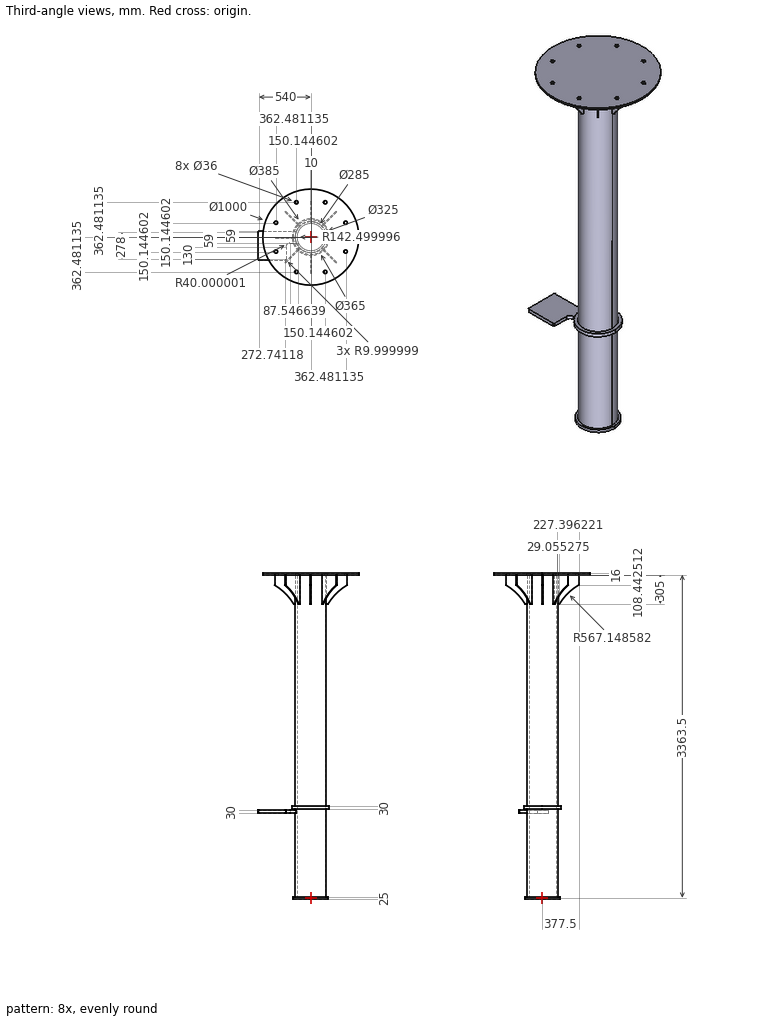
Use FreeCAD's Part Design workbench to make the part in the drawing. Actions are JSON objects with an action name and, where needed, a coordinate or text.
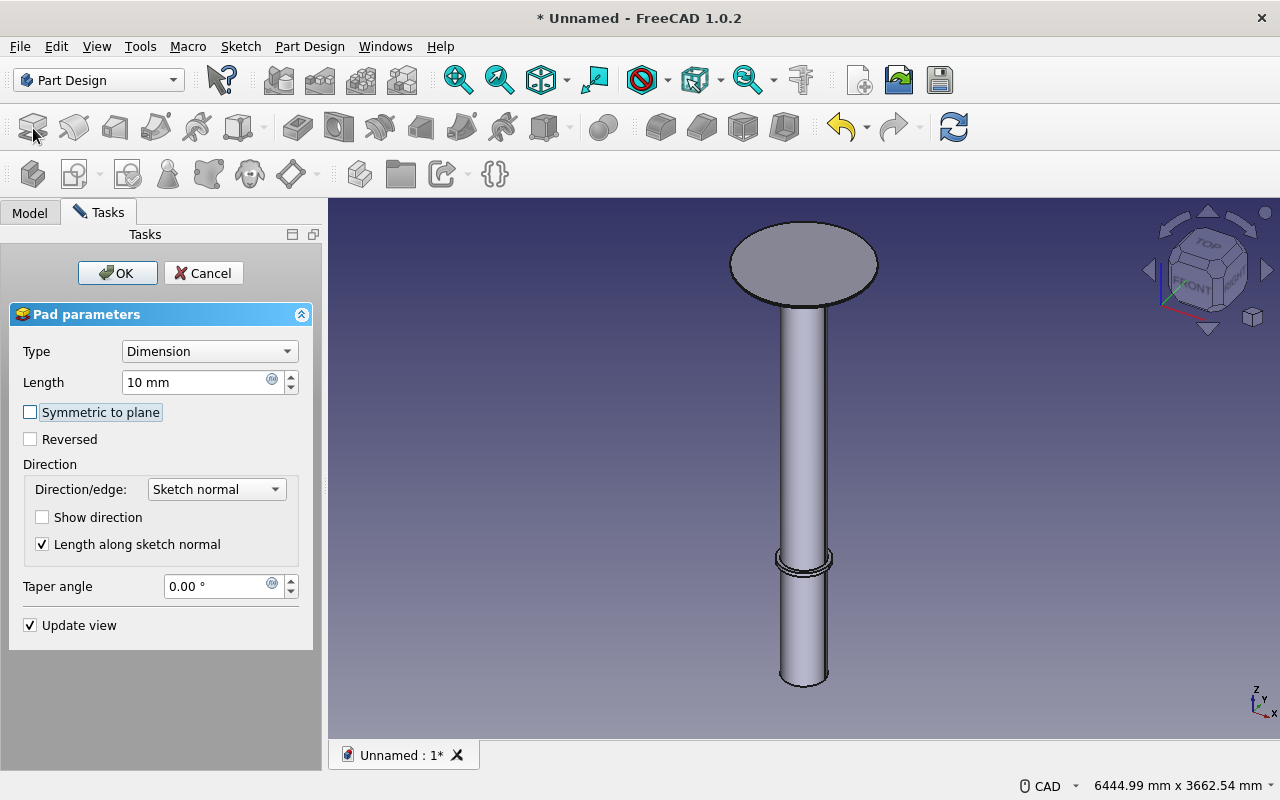
{"action": "left_click", "coordinate": [31, 412]}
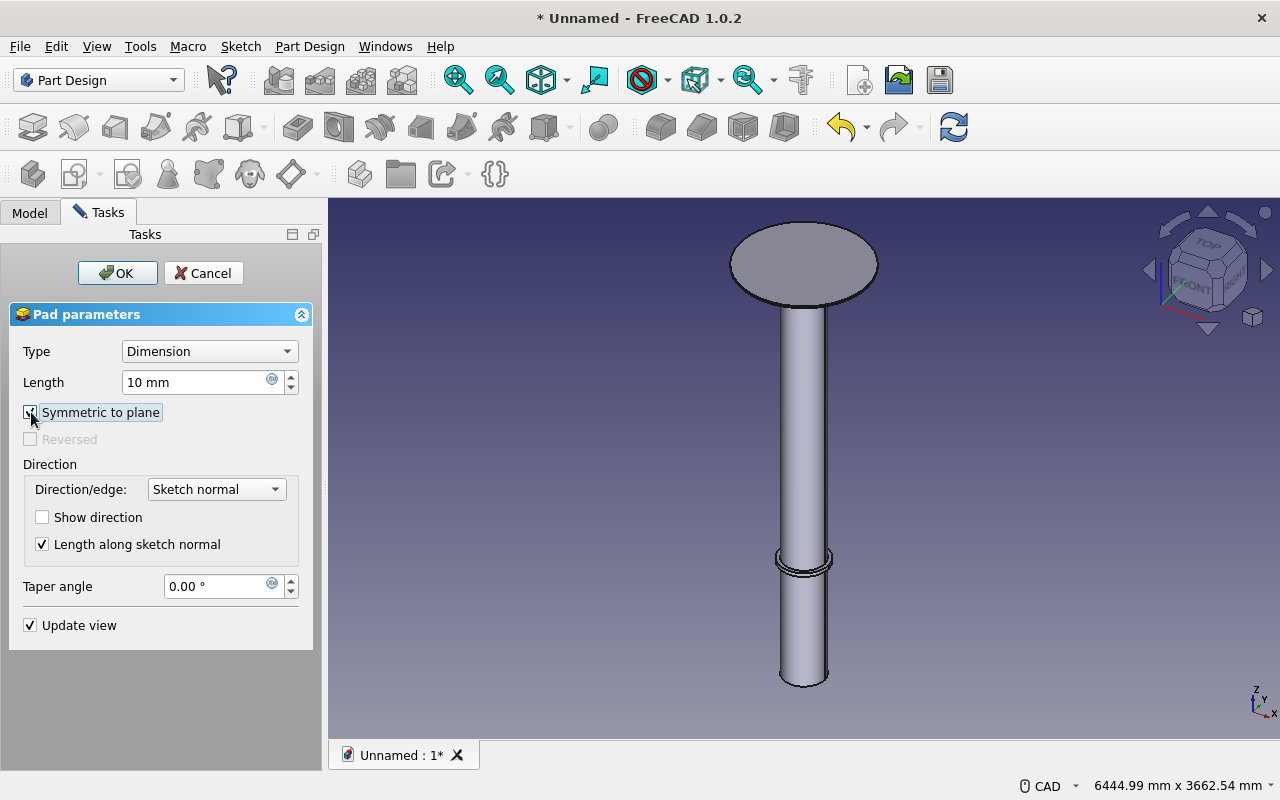
{"action": "left_click", "coordinate": [118, 273]}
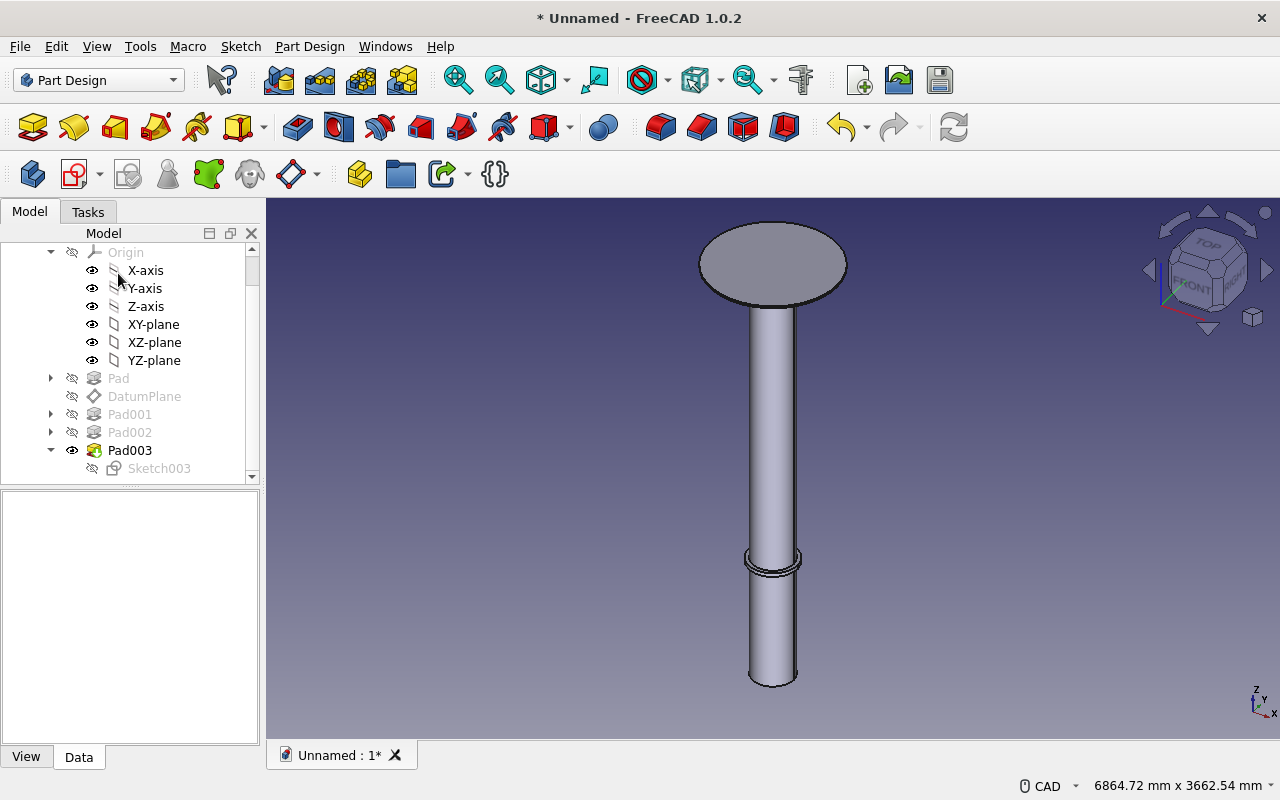
{"action": "left_click", "coordinate": [117, 450]}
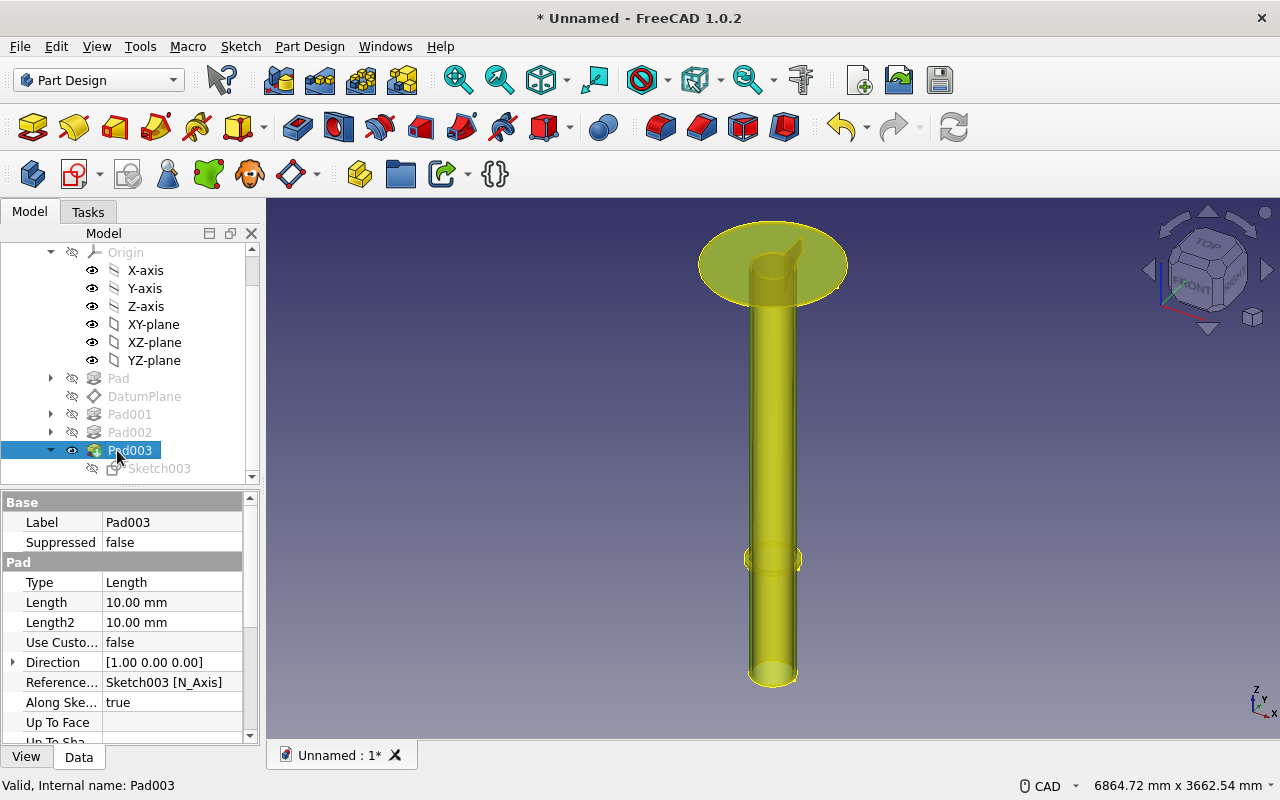
{"action": "left_click", "coordinate": [361, 80]}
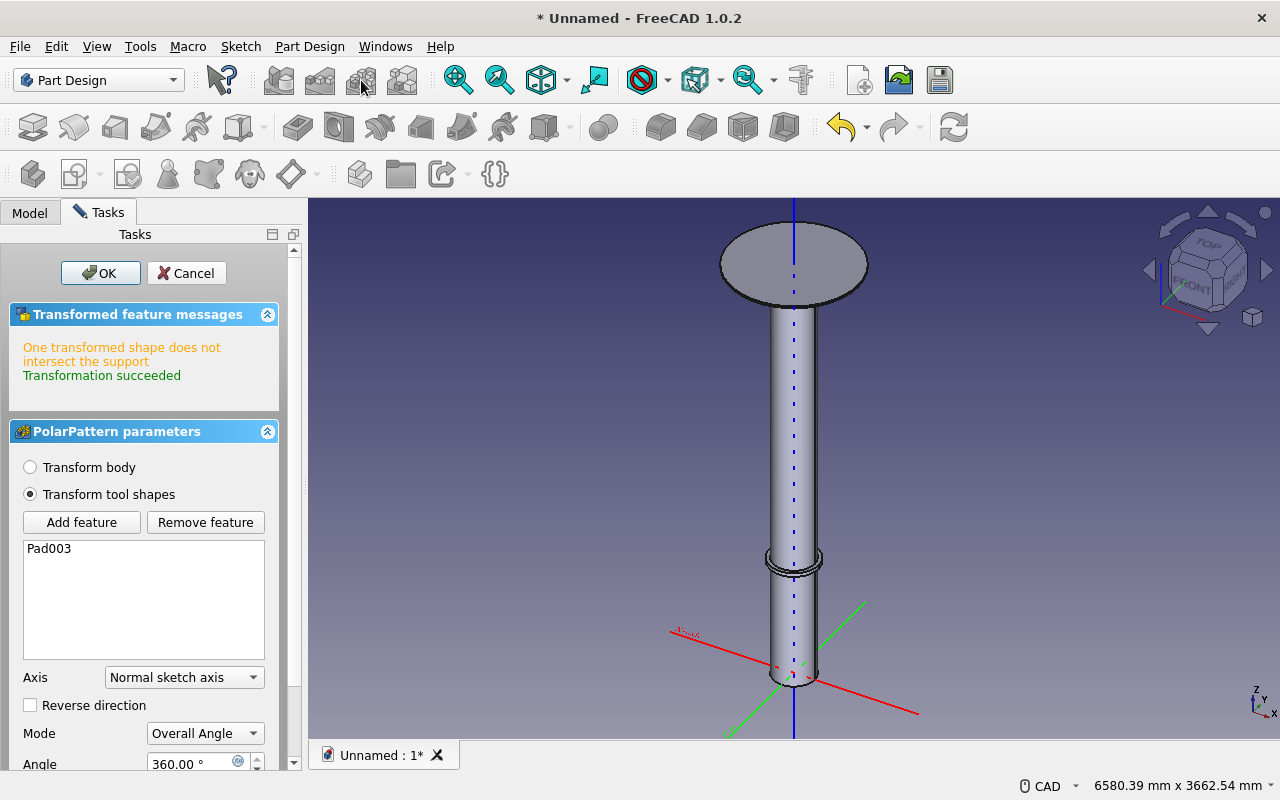
{"action": "left_click", "coordinate": [185, 678]}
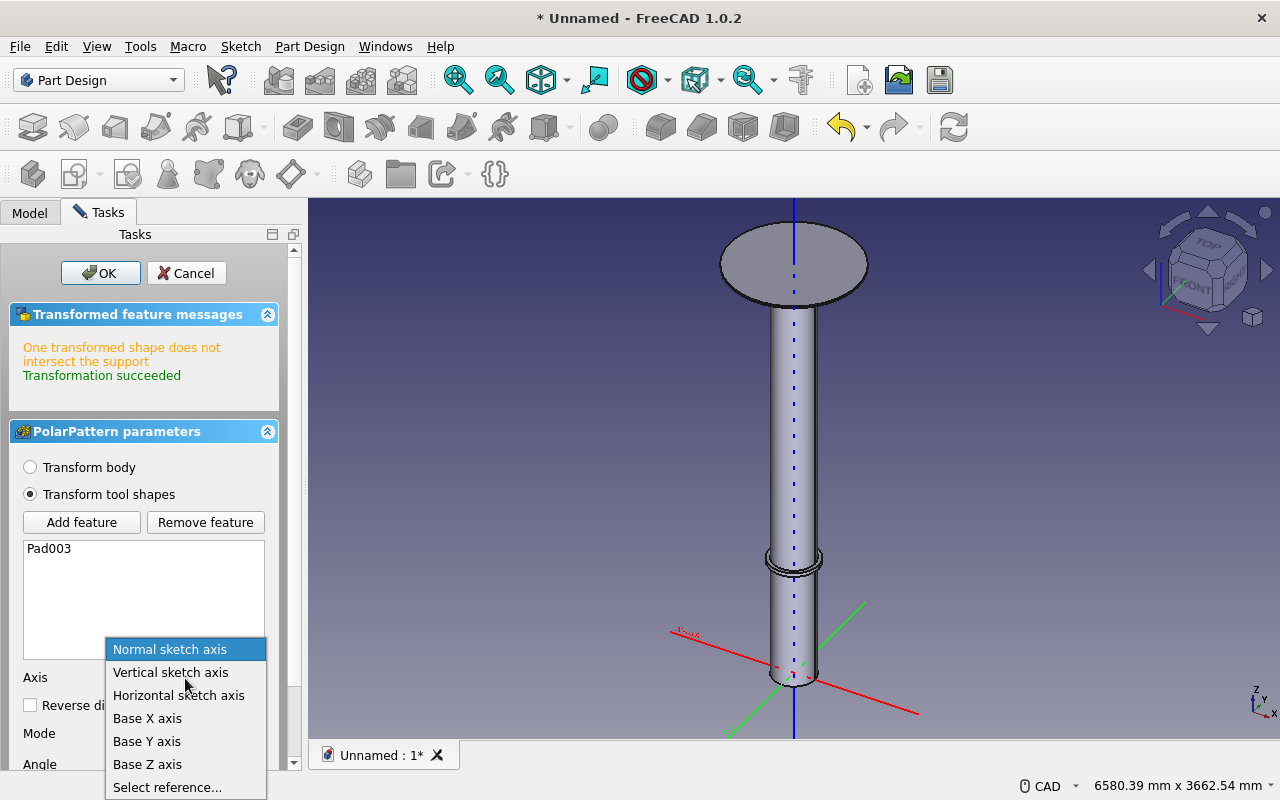
{"action": "left_click", "coordinate": [184, 764]}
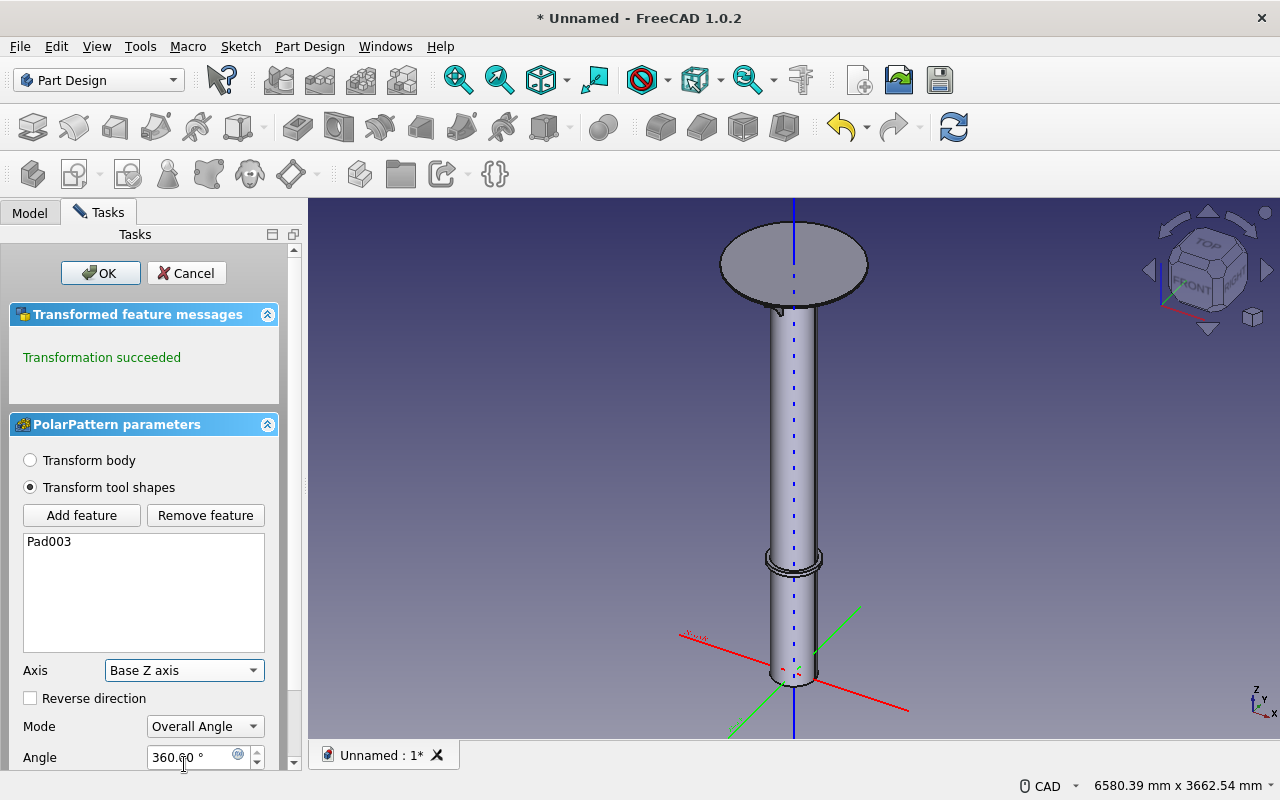
{"action": "scroll", "coordinate": [294, 507], "scroll_direction": "down", "scroll_amount": 2}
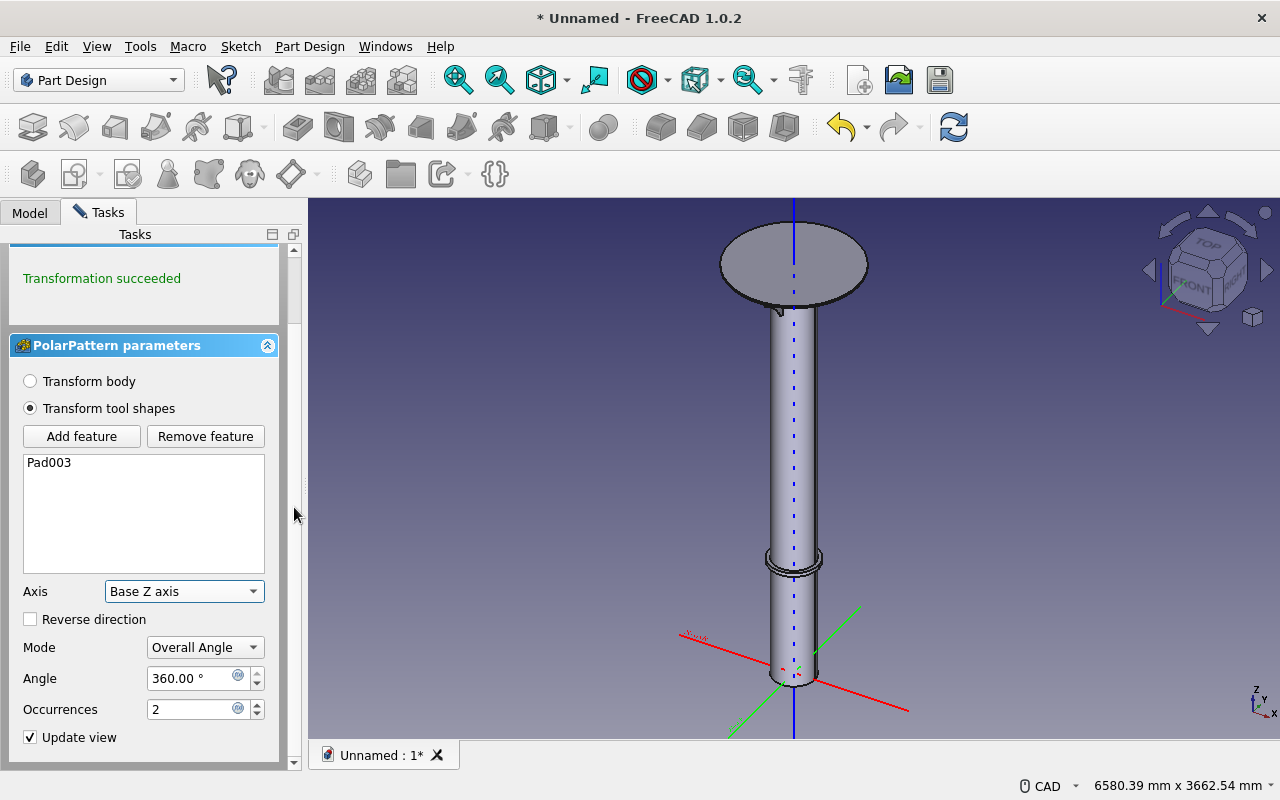
{"action": "triple_click", "coordinate": [199, 710]}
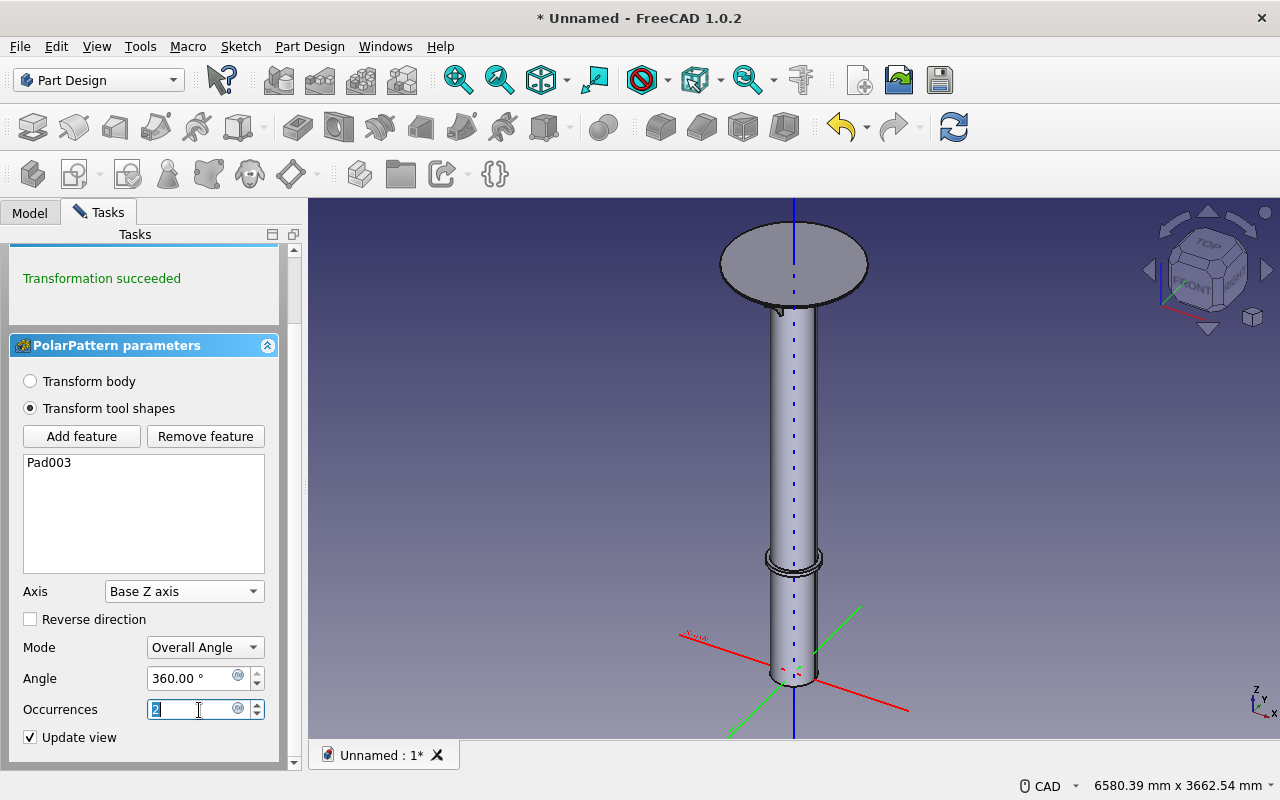
{"action": "type", "text": "8"}
{"action": "key", "text": "Tab"}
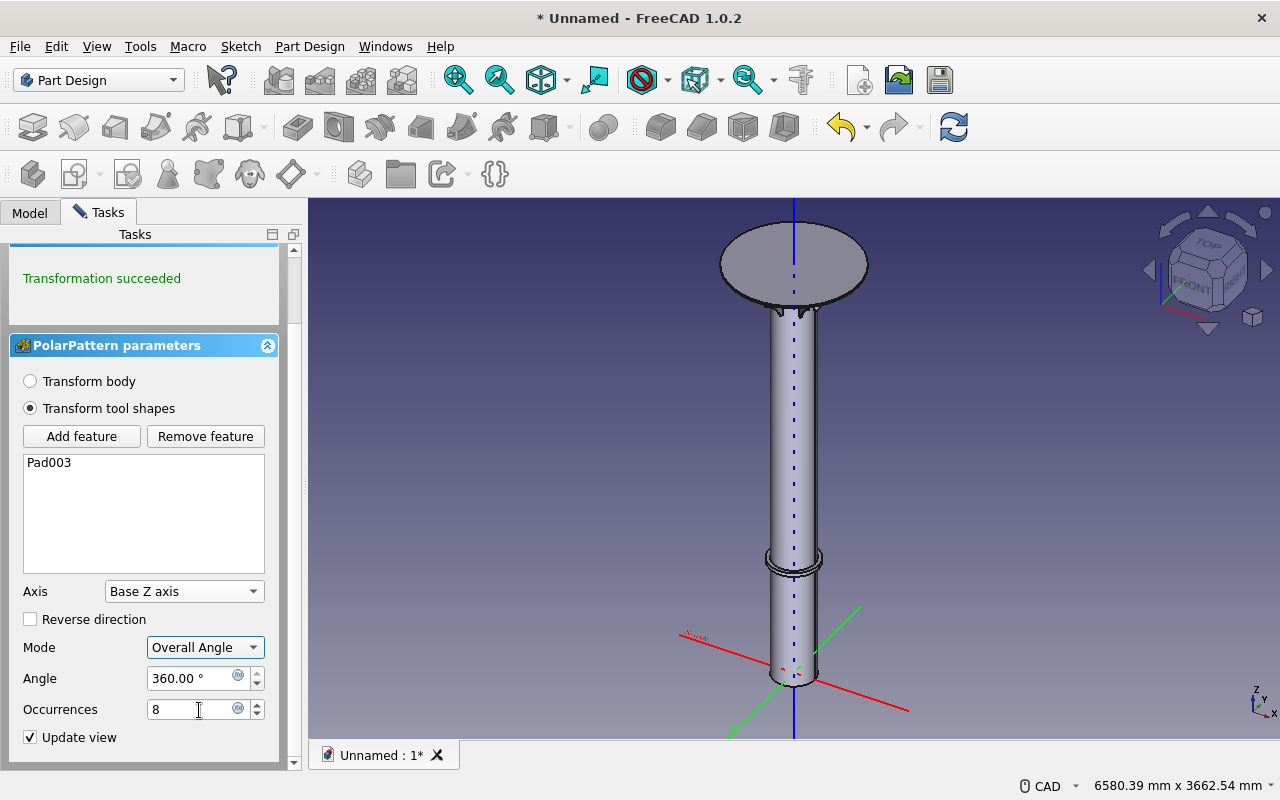
{"action": "scroll", "coordinate": [294, 507], "scroll_direction": "up", "scroll_amount": 3}